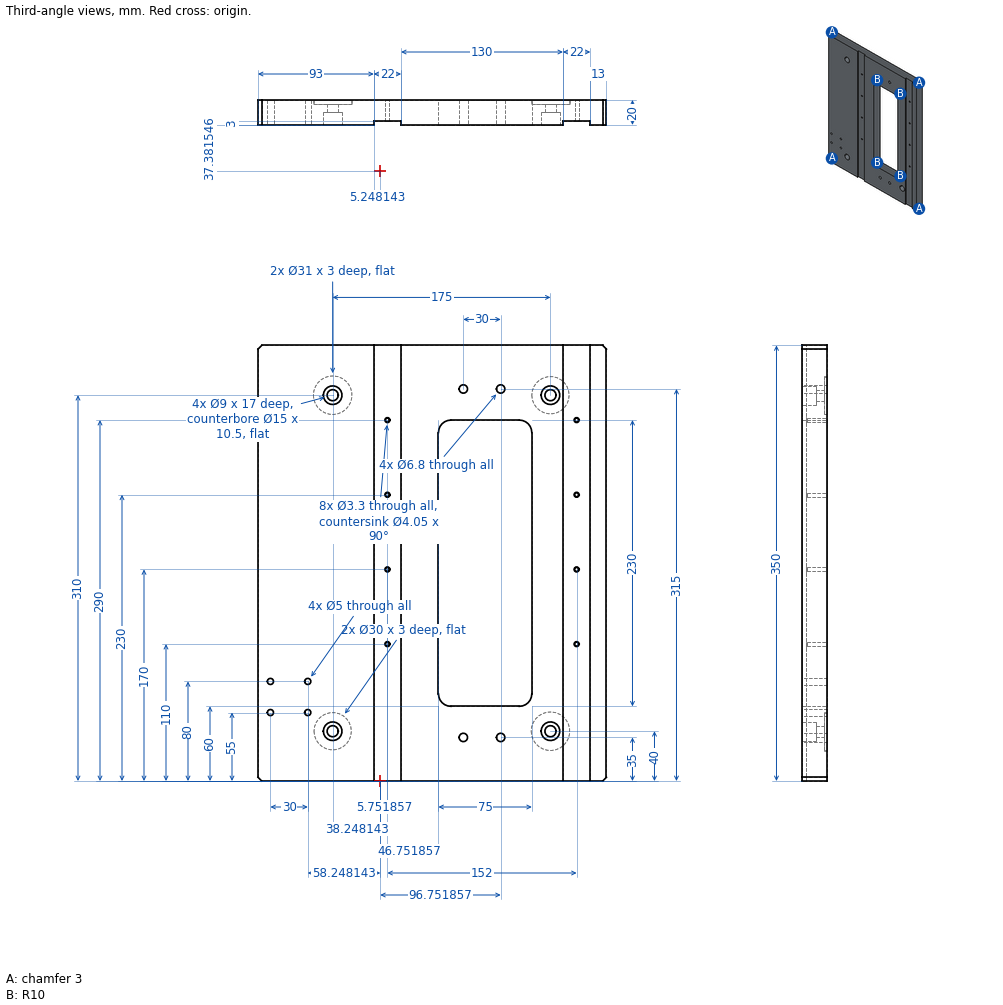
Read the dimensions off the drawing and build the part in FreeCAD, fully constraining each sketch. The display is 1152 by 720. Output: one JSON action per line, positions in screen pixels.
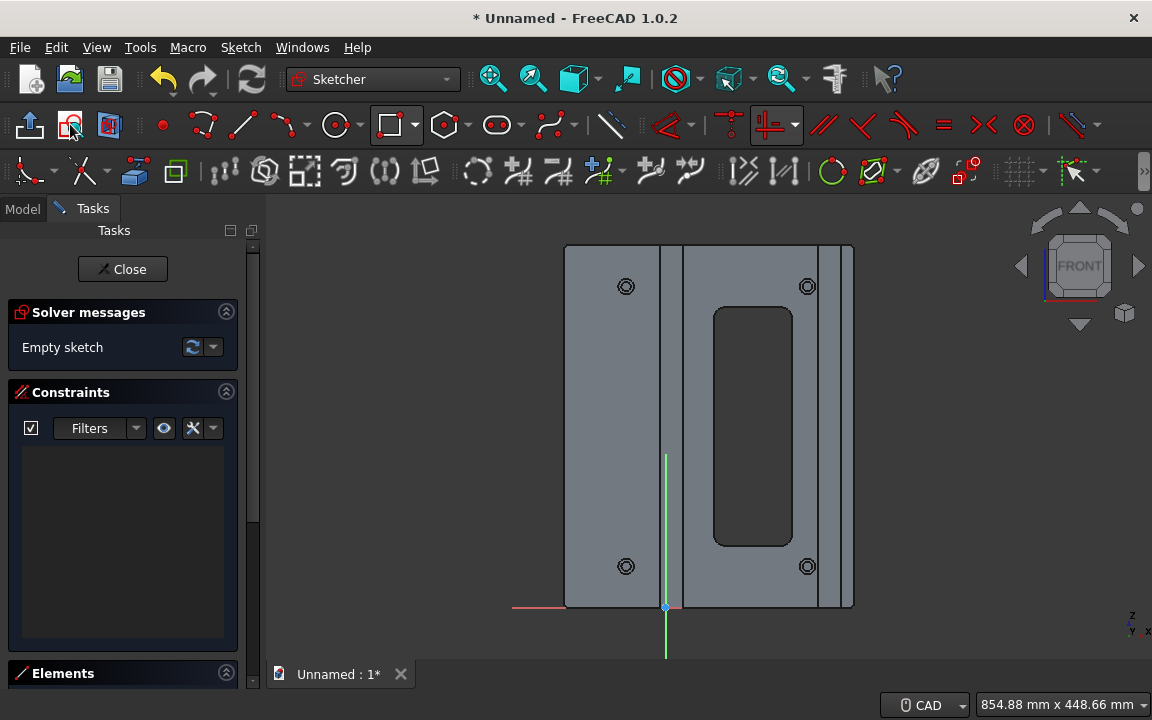
{"action": "scroll", "coordinate": [294, 290], "scroll_direction": "down", "scroll_amount": 1}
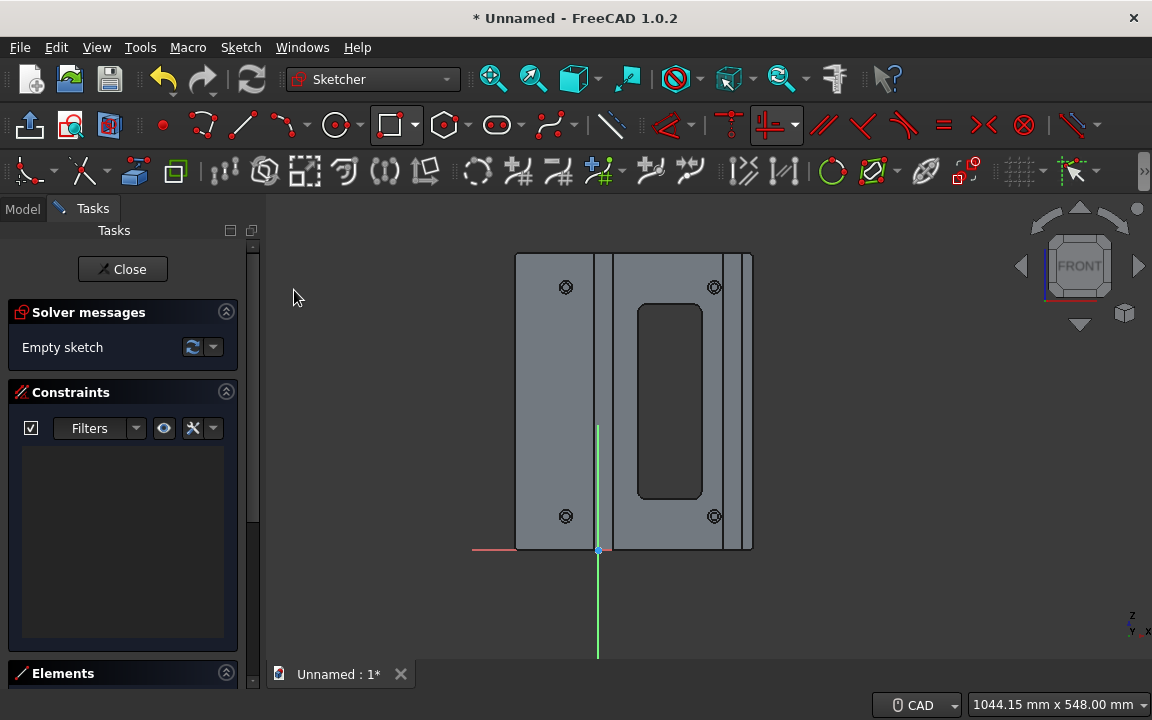
{"action": "left_click", "coordinate": [336, 126]}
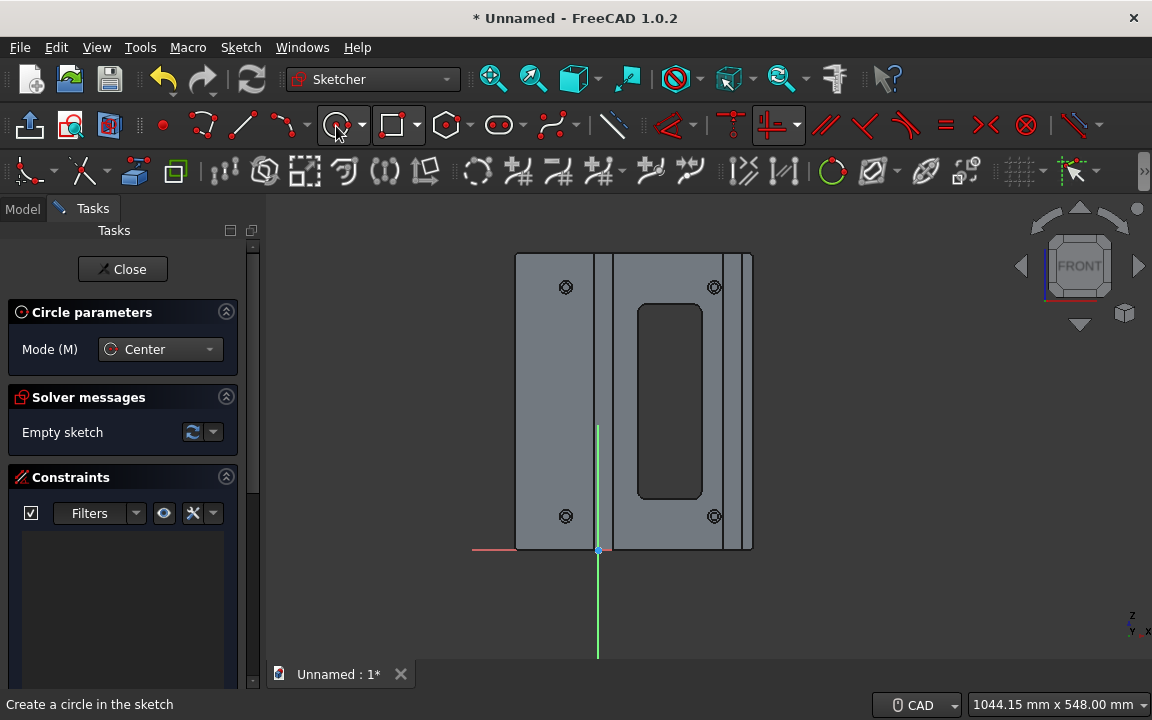
{"action": "scroll", "coordinate": [603, 304], "scroll_direction": "up", "scroll_amount": 14}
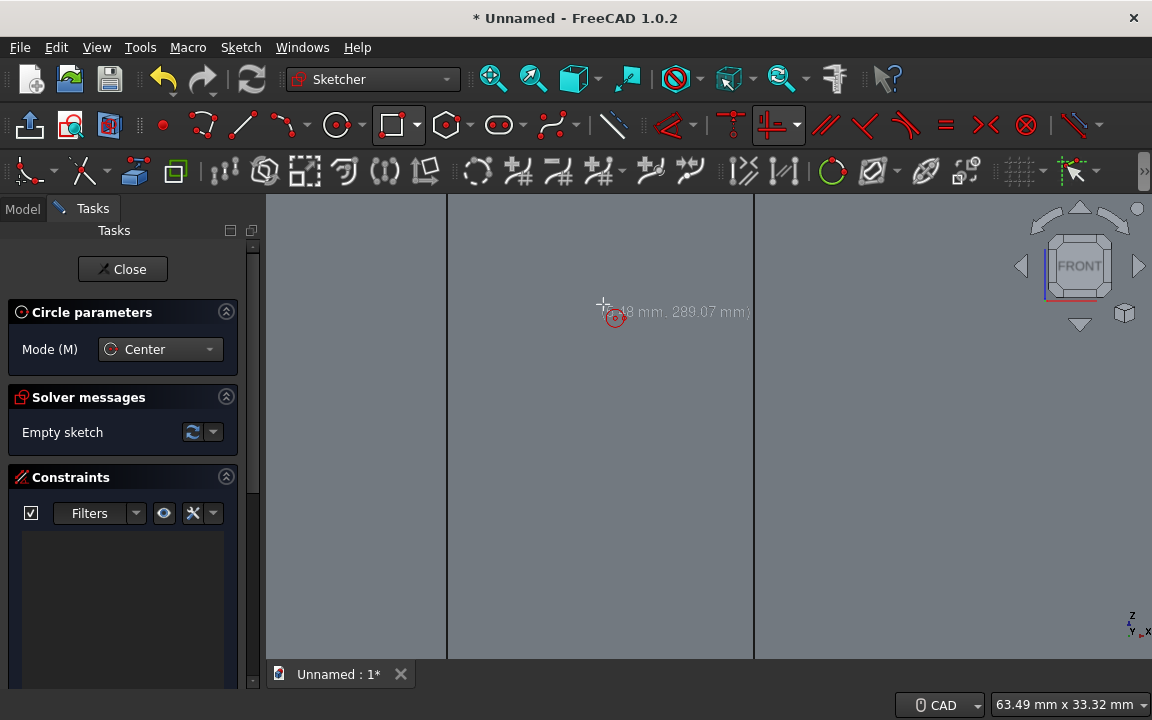
{"action": "scroll", "coordinate": [561, 275], "scroll_direction": "down", "scroll_amount": 13}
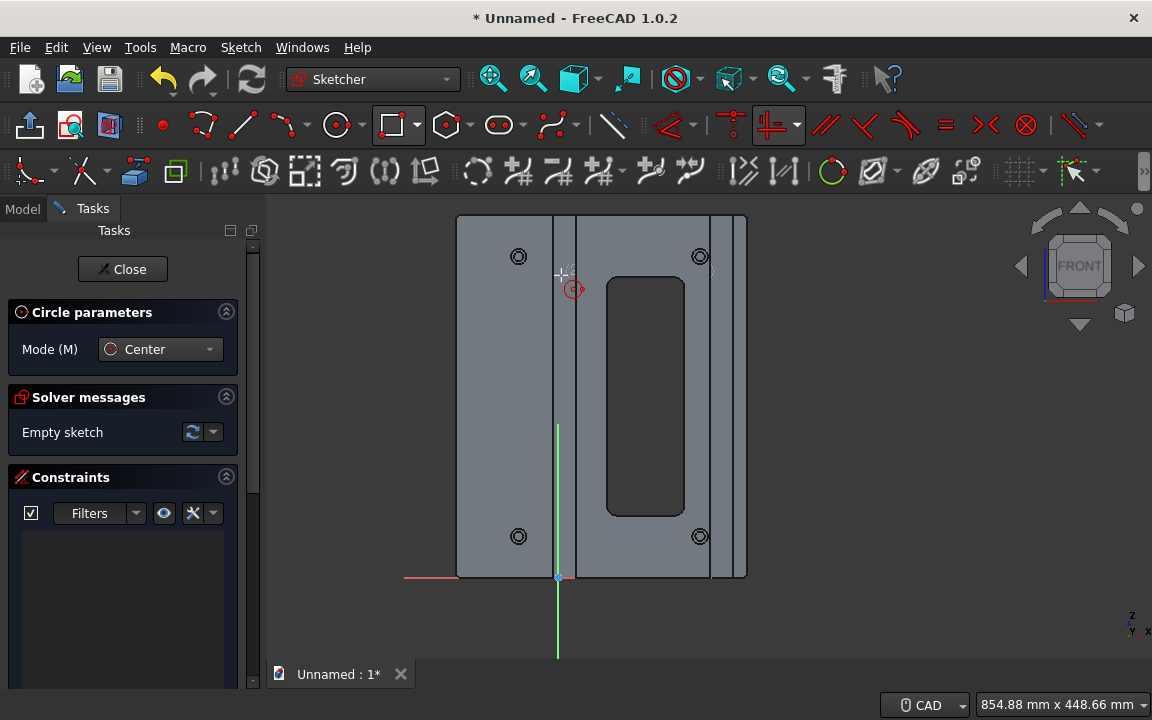
{"action": "scroll", "coordinate": [564, 277], "scroll_direction": "up", "scroll_amount": 5}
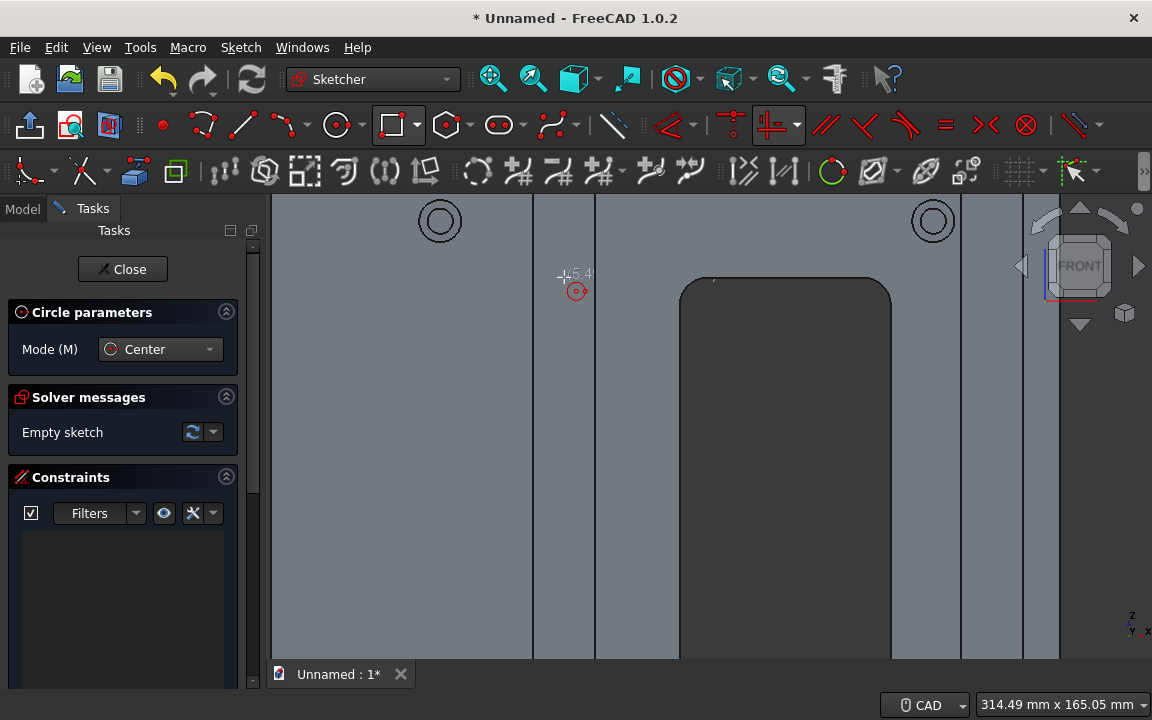
{"action": "left_click", "coordinate": [564, 278]}
{"action": "mouse_move", "coordinate": [567, 274]}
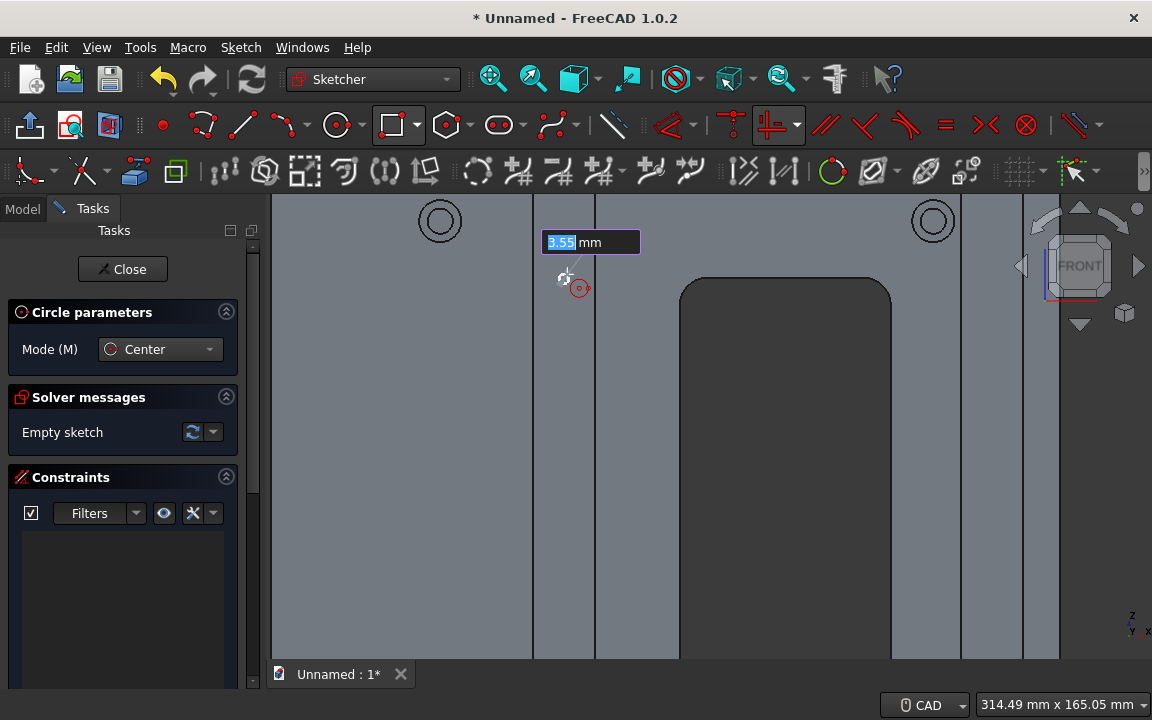
{"action": "type", "text": "3.3"}
{"action": "key", "text": "Return"}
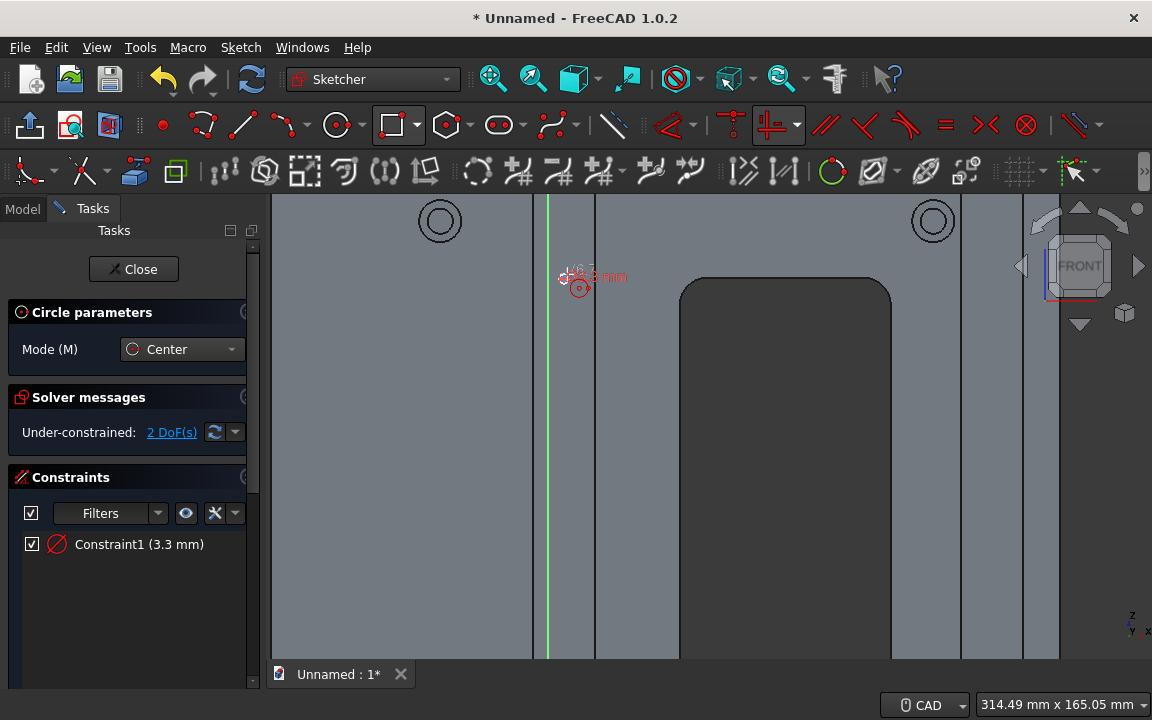
{"action": "scroll", "coordinate": [564, 447], "scroll_direction": "up", "scroll_amount": 8}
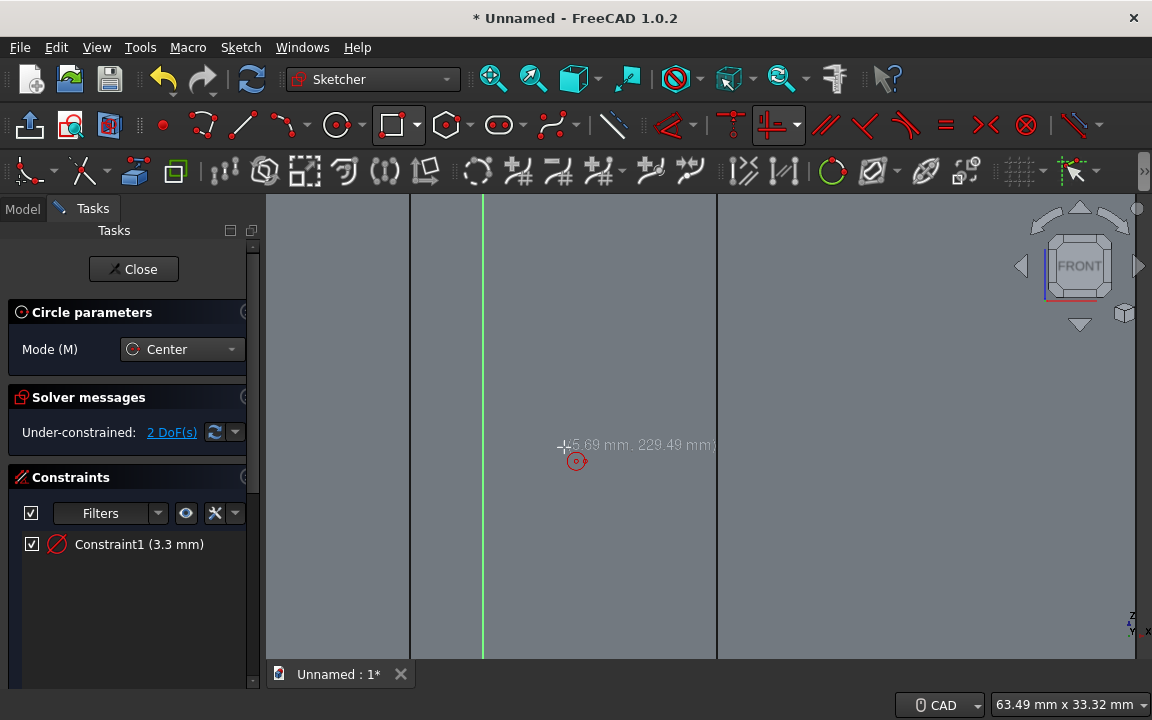
{"action": "scroll", "coordinate": [564, 331], "scroll_direction": "down", "scroll_amount": 13}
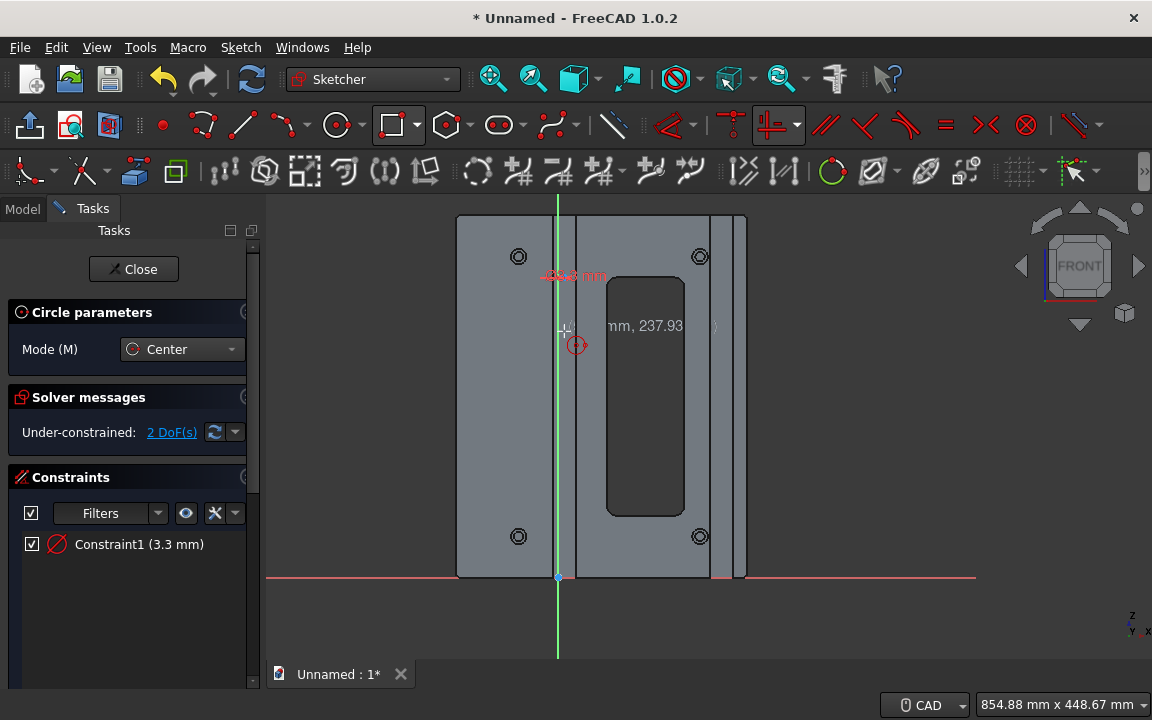
{"action": "scroll", "coordinate": [564, 340], "scroll_direction": "up", "scroll_amount": 5}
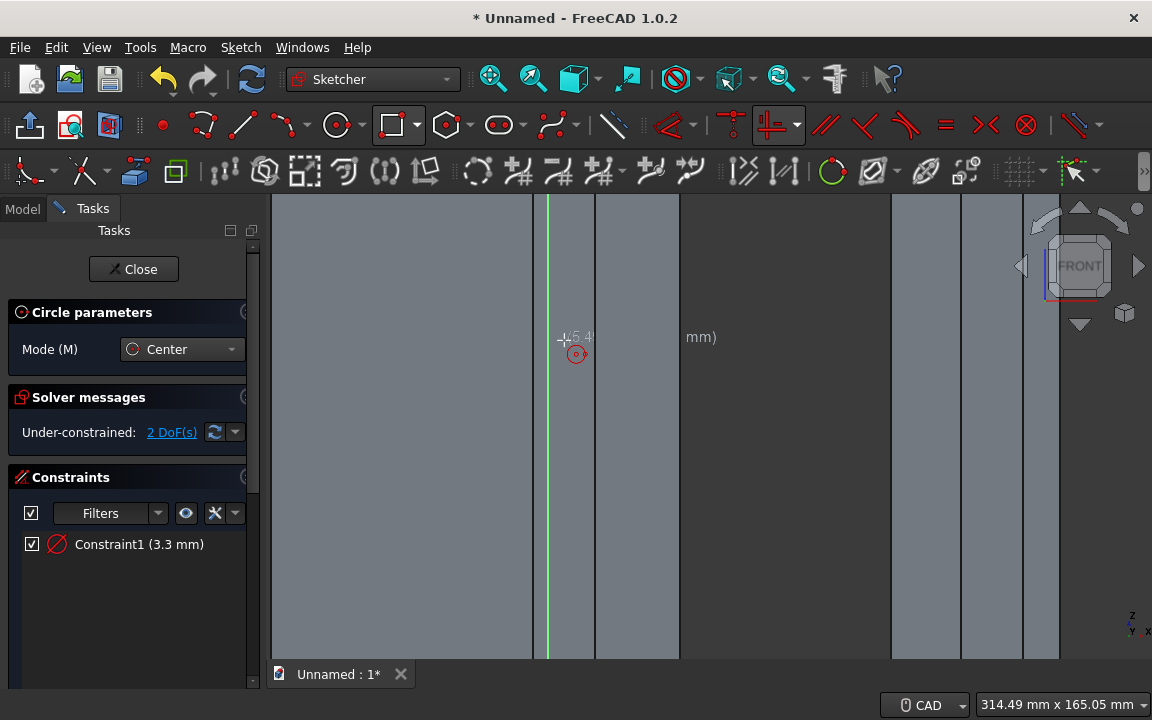
{"action": "left_click", "coordinate": [564, 338]}
{"action": "mouse_move", "coordinate": [567, 335]}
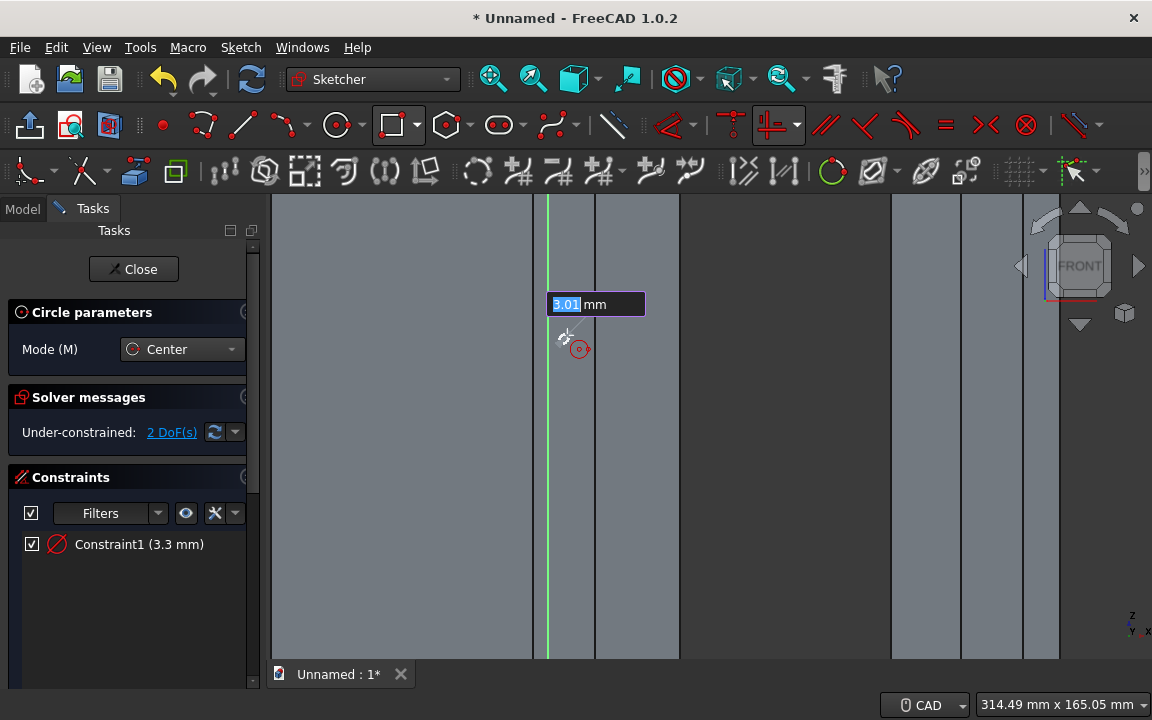
{"action": "type", "text": "3.3"}
{"action": "key", "text": "Return"}